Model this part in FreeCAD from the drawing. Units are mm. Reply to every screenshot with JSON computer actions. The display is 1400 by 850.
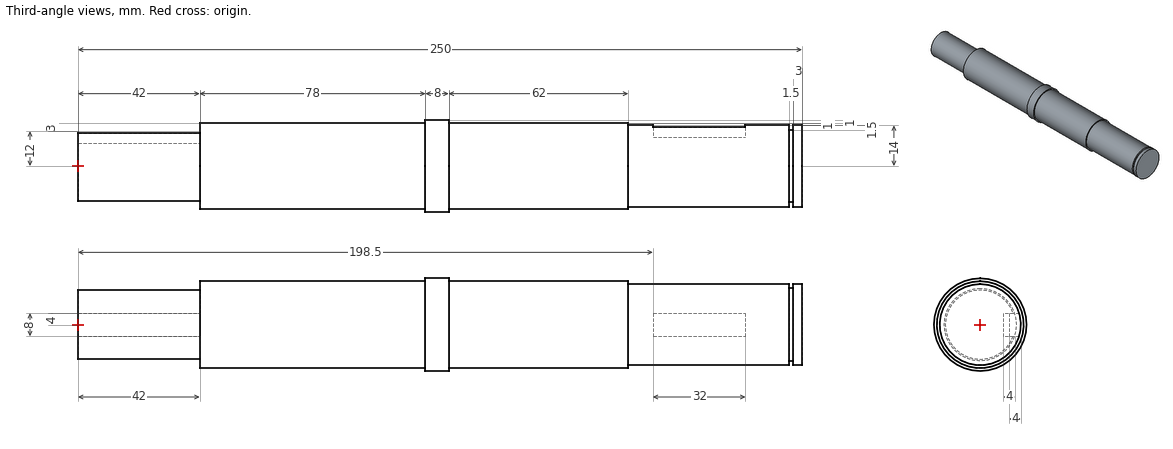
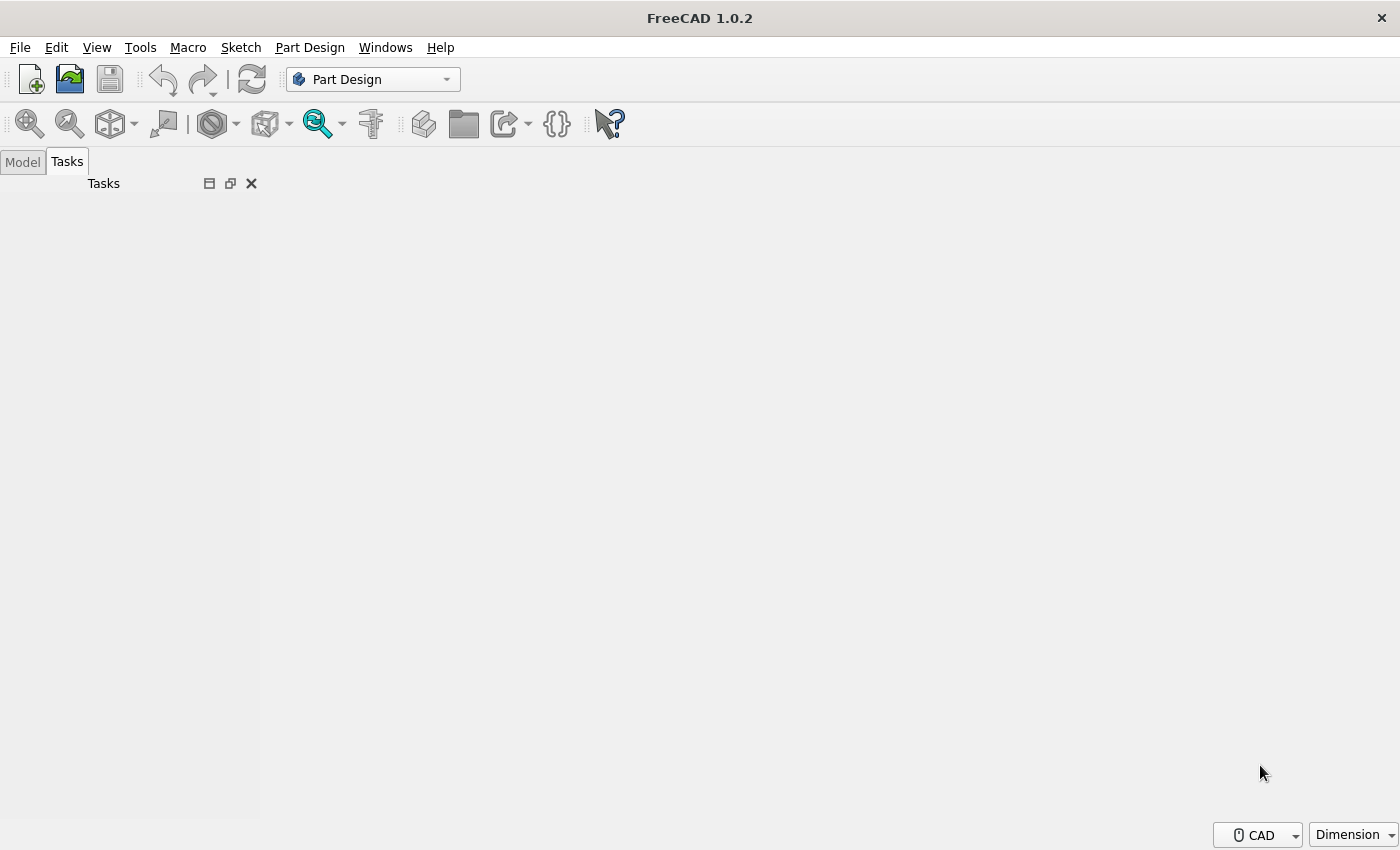
{"action": "left_click", "coordinate": [478, 124]}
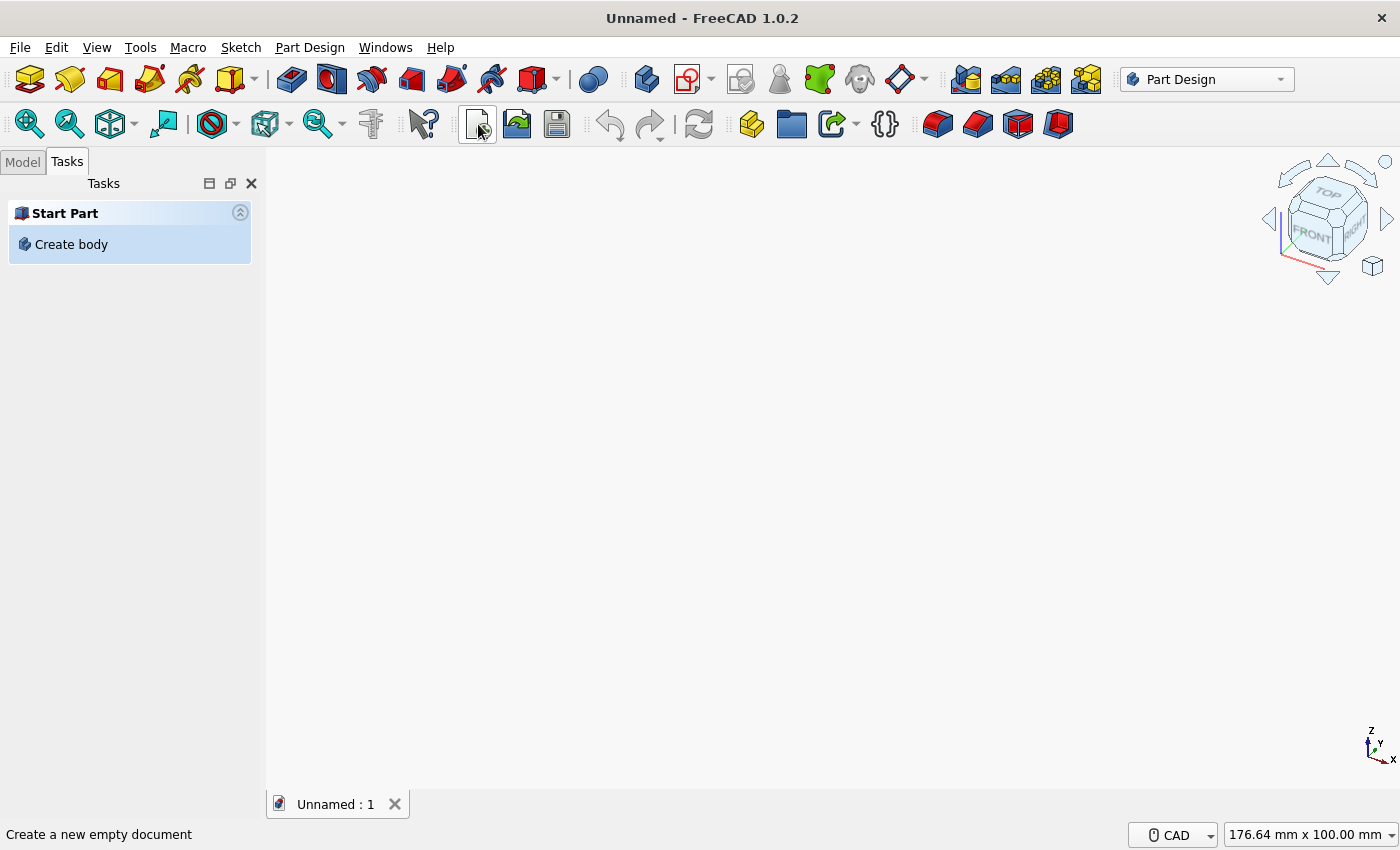
{"action": "left_click", "coordinate": [688, 80]}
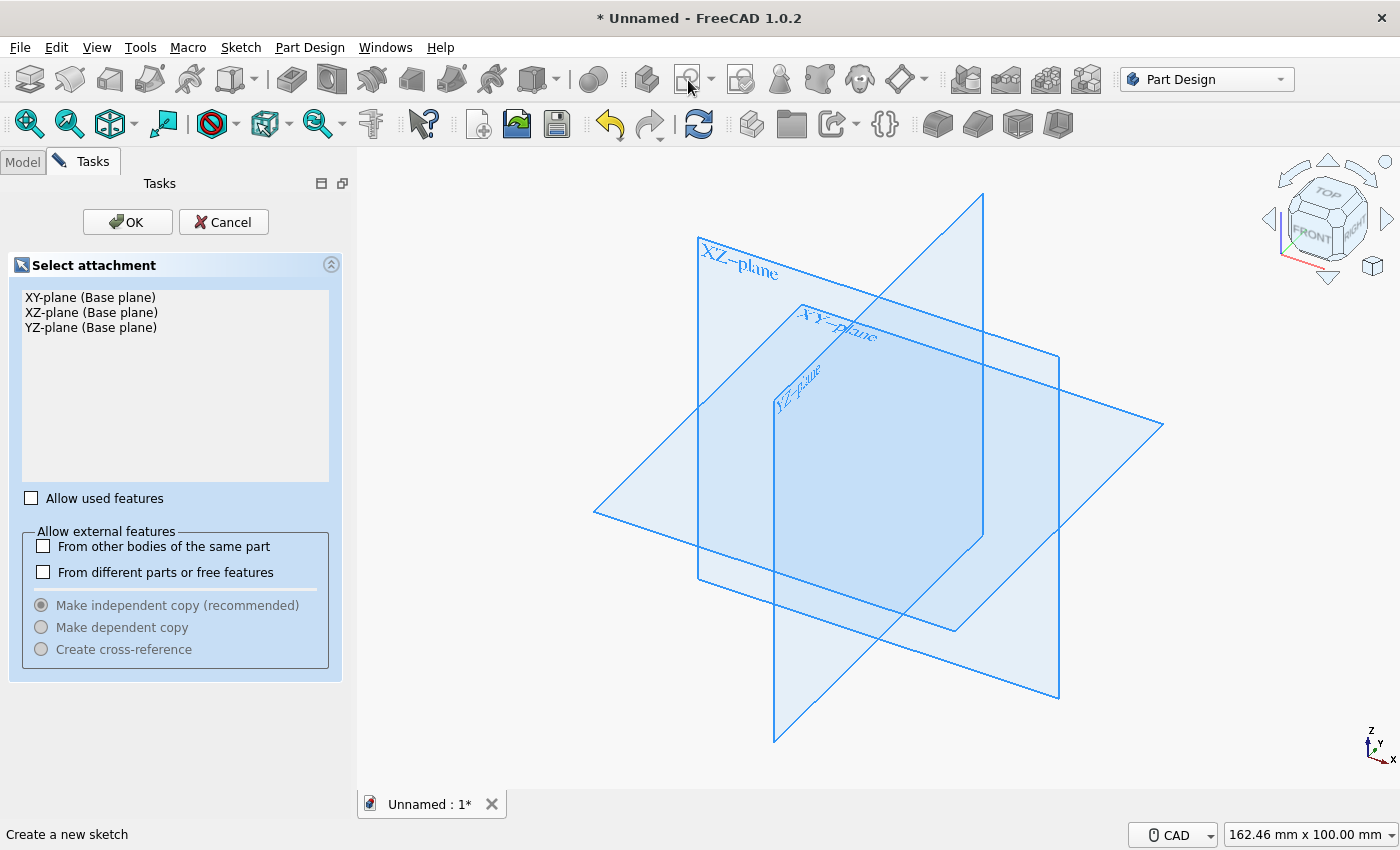
{"action": "left_click", "coordinate": [82, 298]}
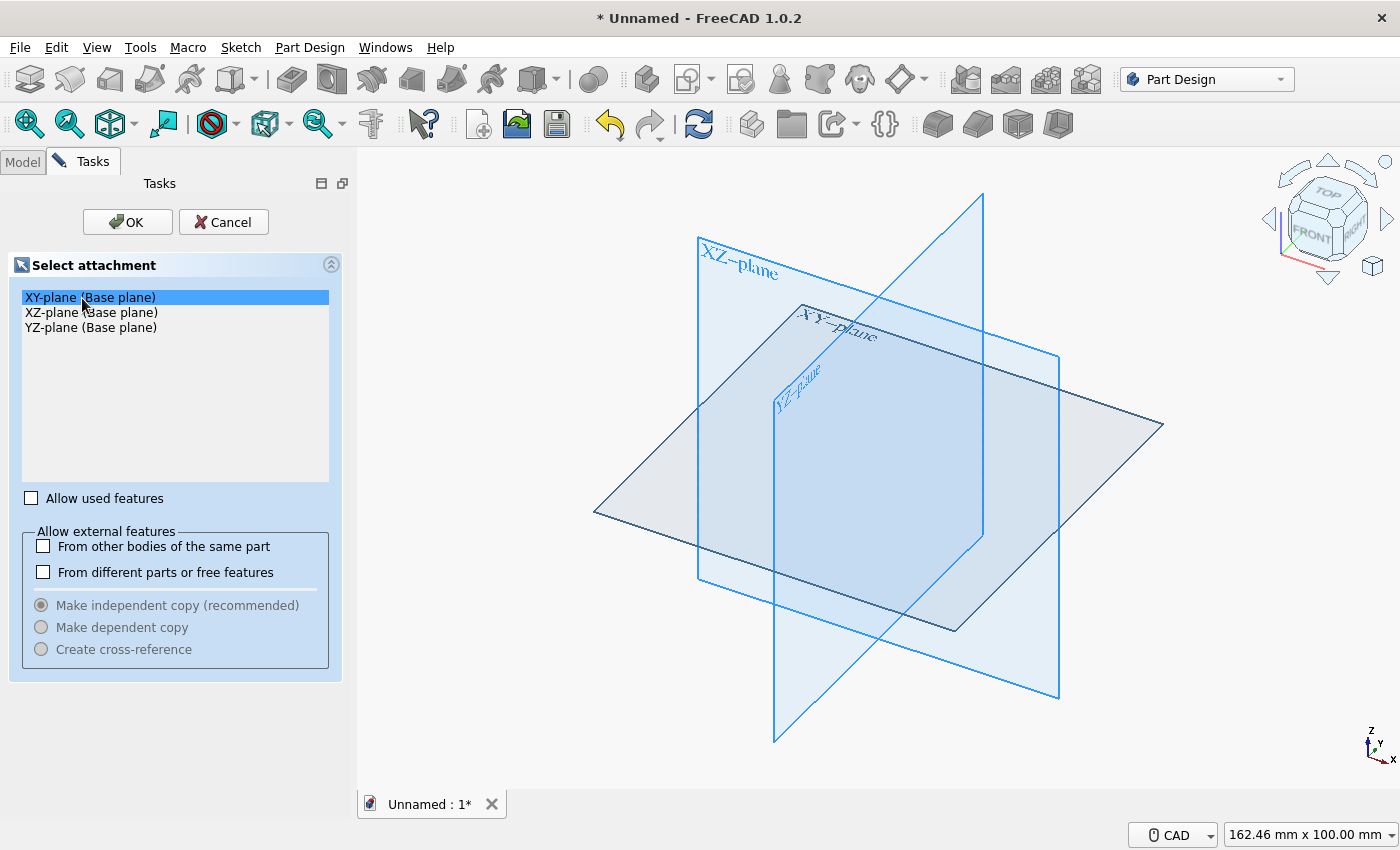
{"action": "left_click", "coordinate": [128, 222]}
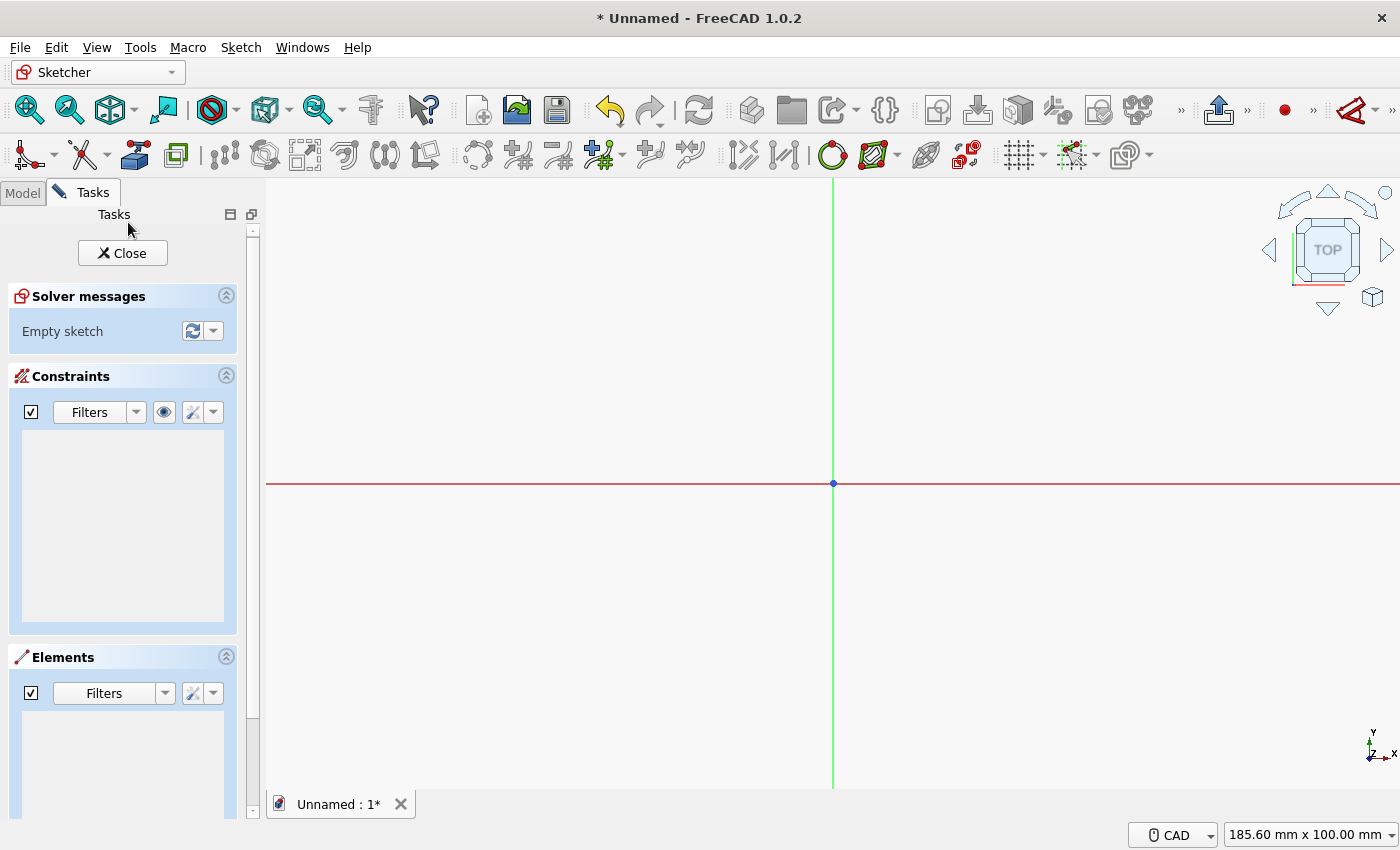
{"action": "scroll", "coordinate": [294, 512], "scroll_direction": "down", "scroll_amount": 5}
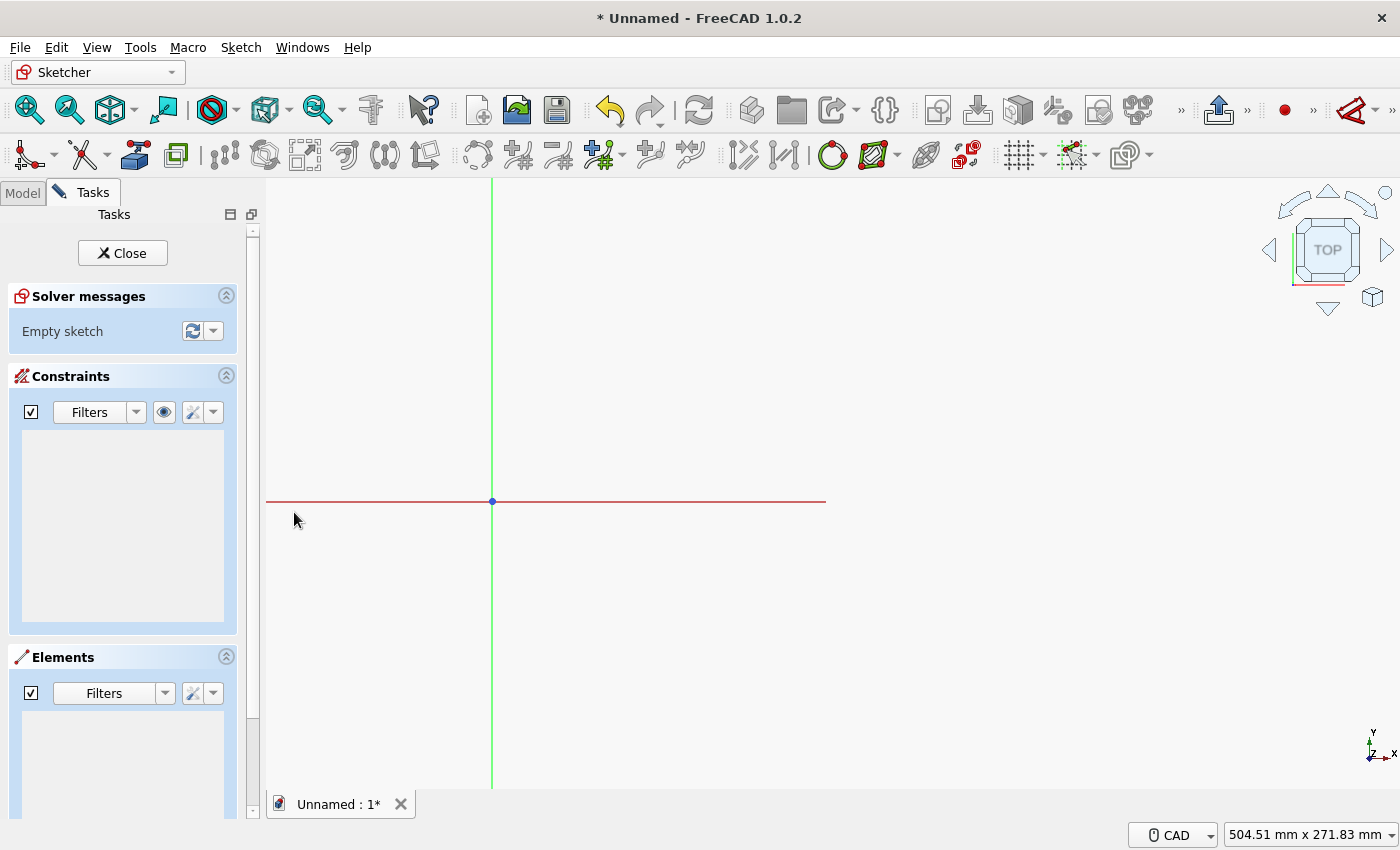
{"action": "key", "text": "g m"}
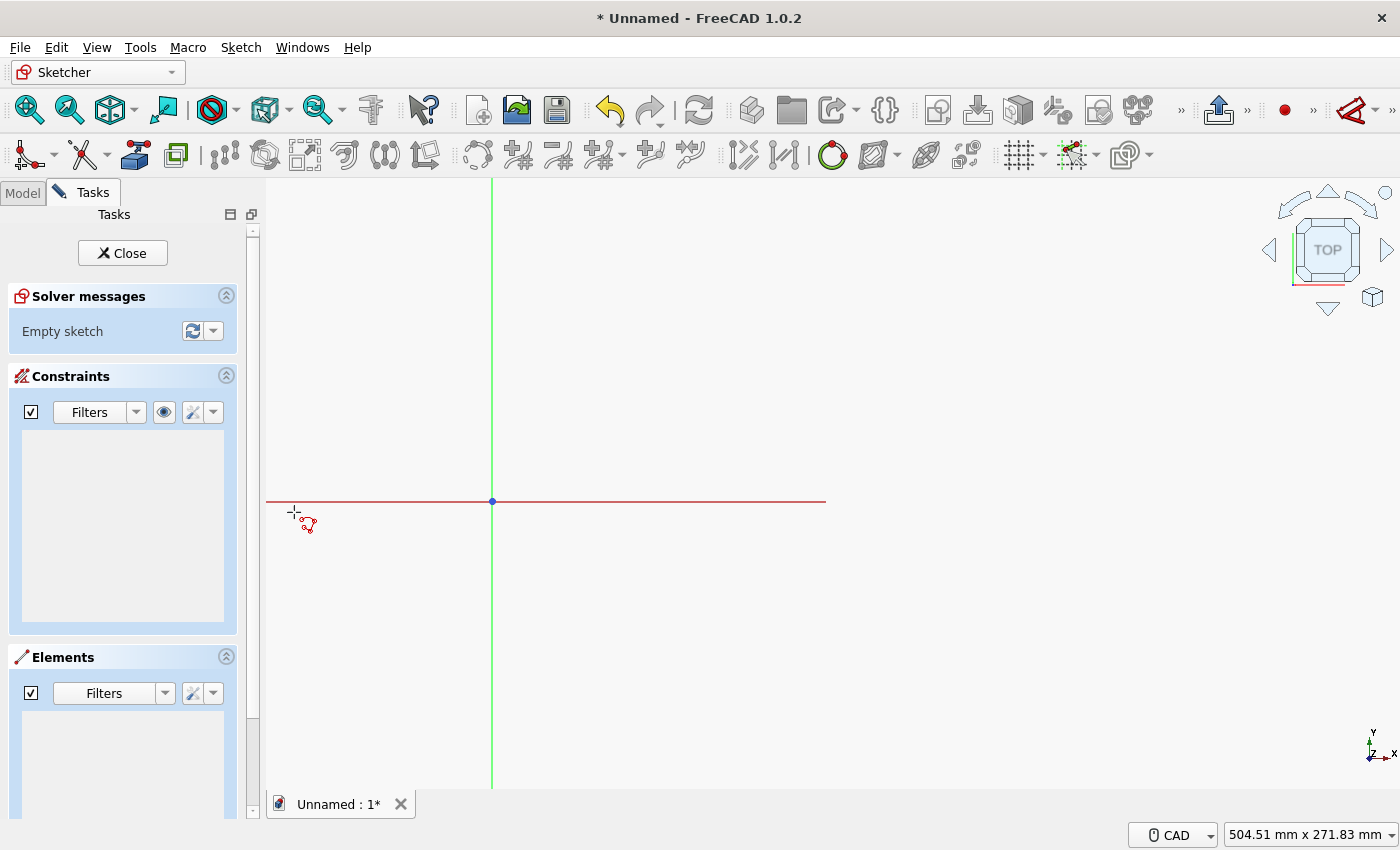
{"action": "left_click", "coordinate": [492, 502]}
{"action": "left_click", "coordinate": [1054, 493]}
{"action": "left_click", "coordinate": [1054, 470]}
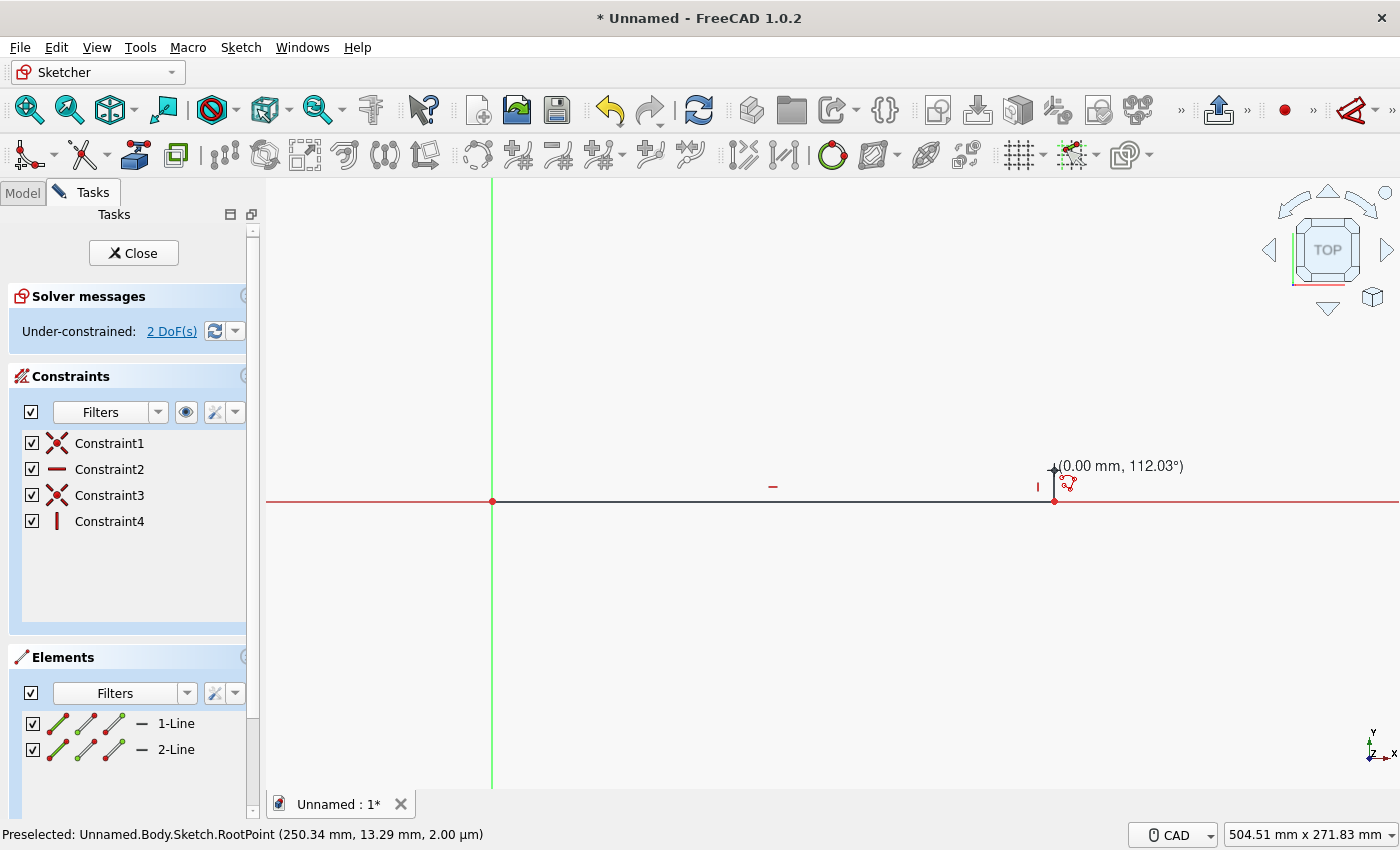
{"action": "scroll", "coordinate": [1047, 470], "scroll_direction": "up", "scroll_amount": 5}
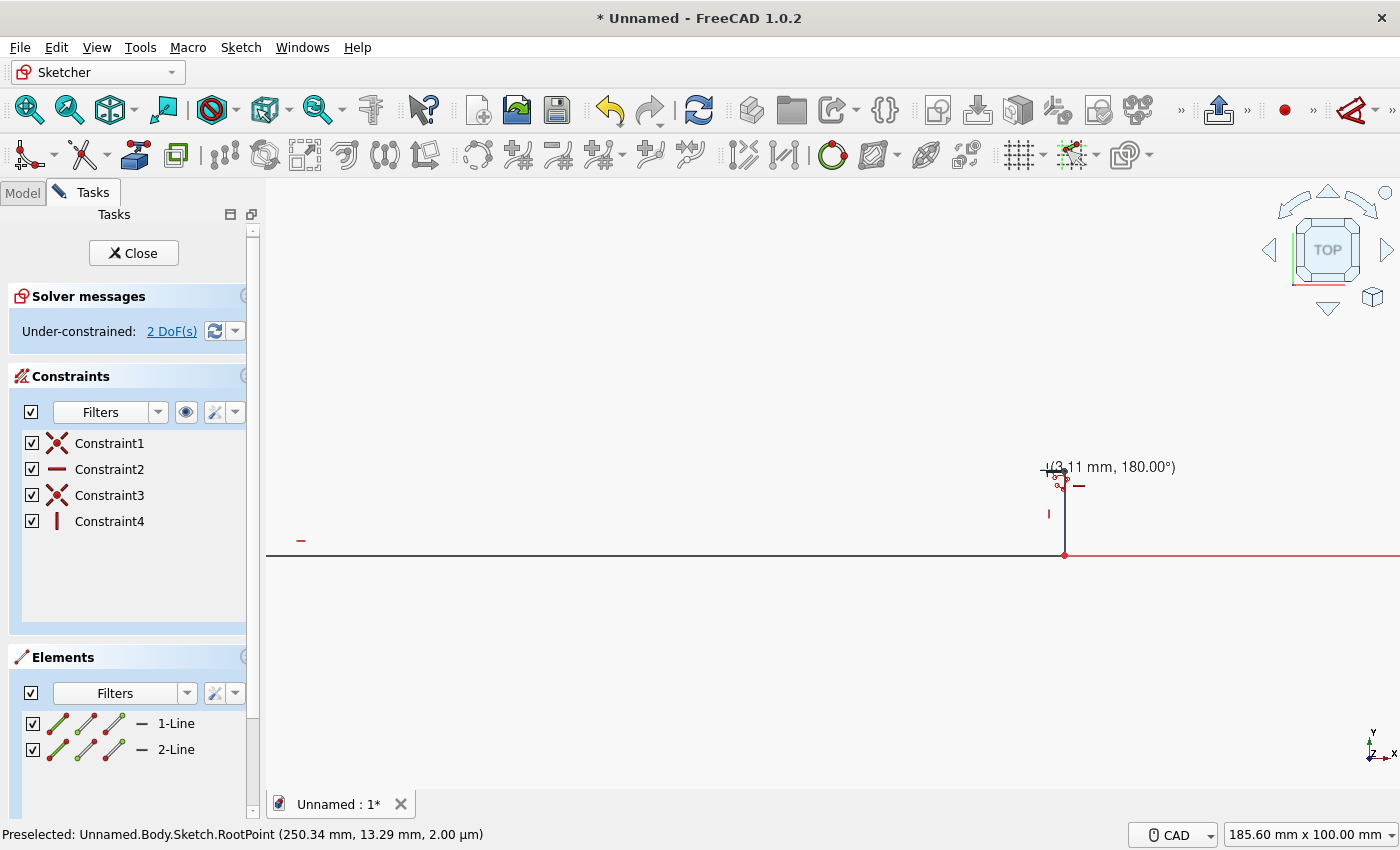
{"action": "left_click", "coordinate": [1047, 469]}